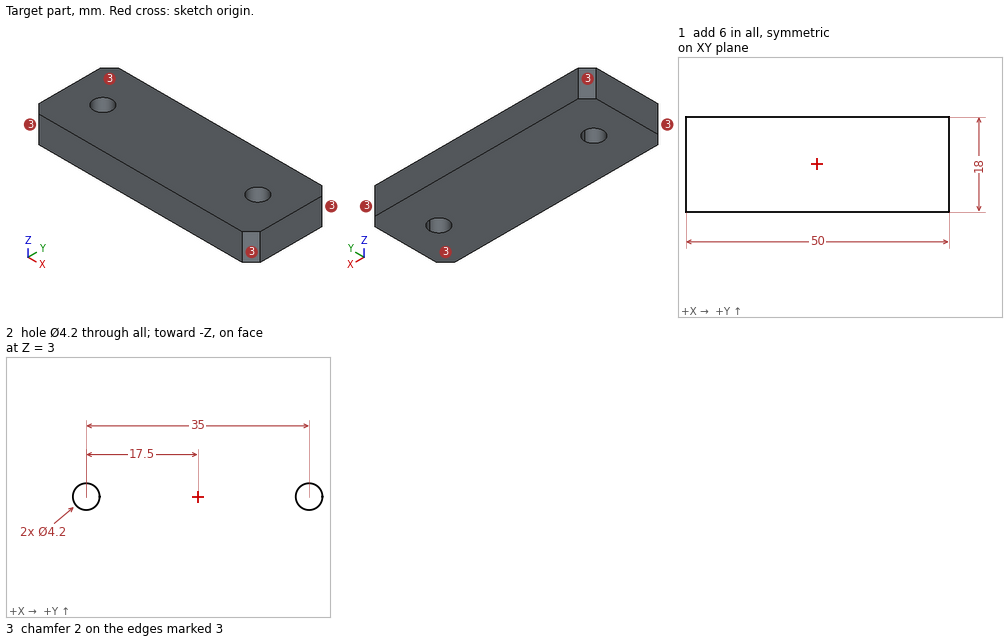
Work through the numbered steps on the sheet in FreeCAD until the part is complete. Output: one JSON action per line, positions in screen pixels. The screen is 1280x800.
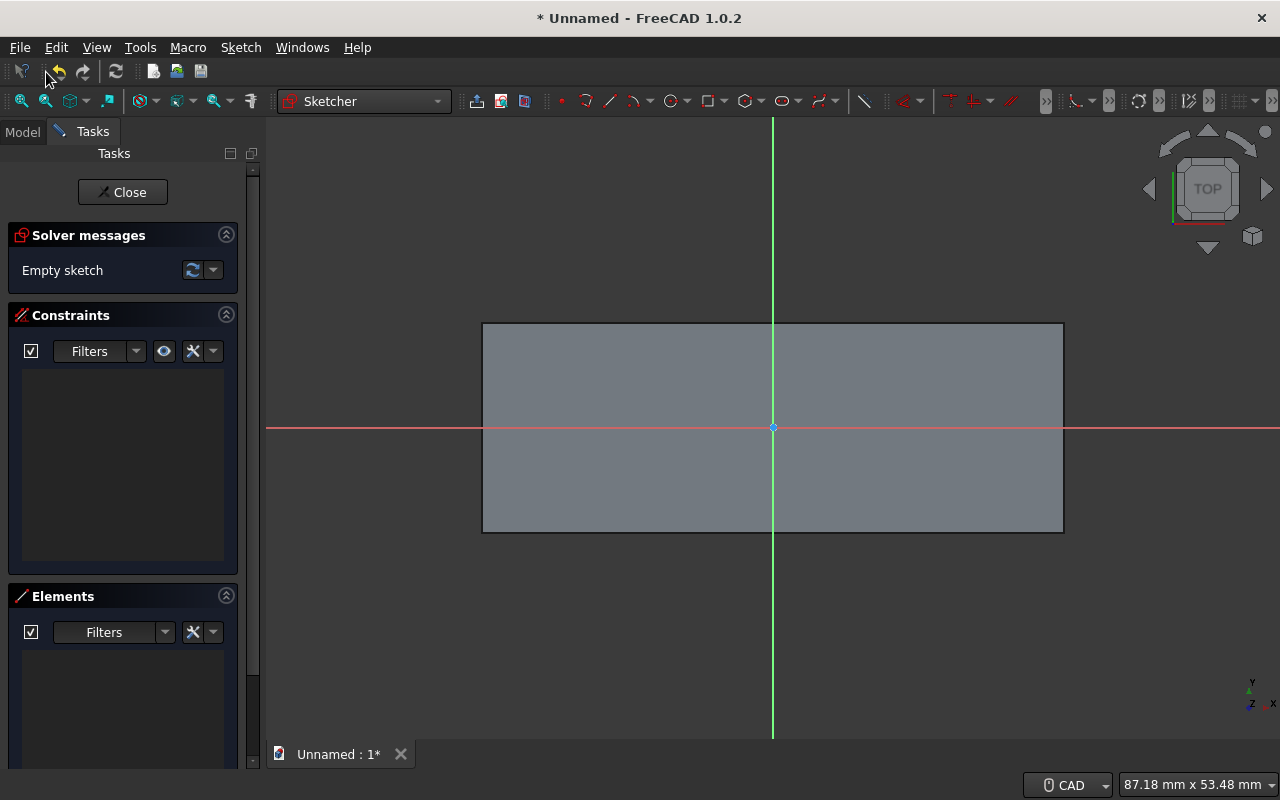
{"action": "key", "text": "g c"}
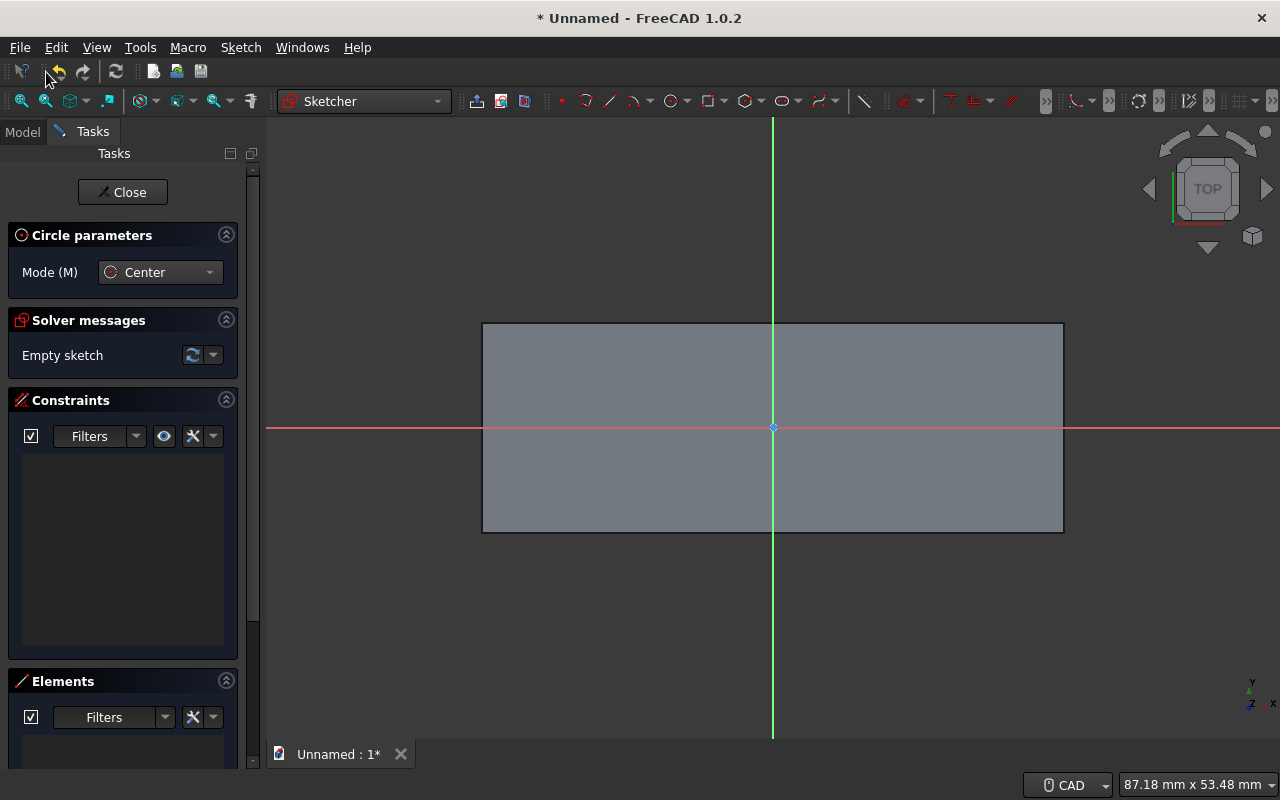
{"action": "left_click", "coordinate": [569, 428]}
{"action": "left_click", "coordinate": [587, 411]}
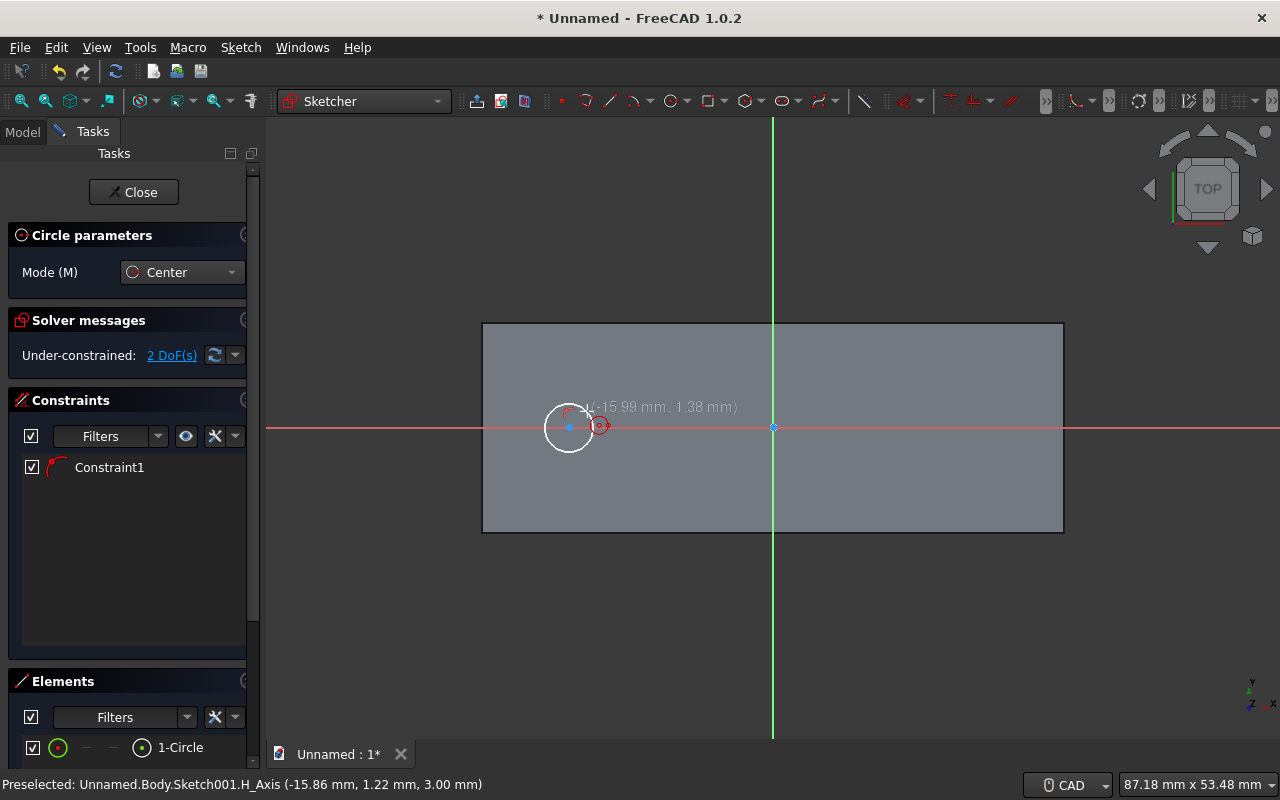
{"action": "left_click", "coordinate": [977, 428]}
{"action": "left_click", "coordinate": [994, 411]}
{"action": "key", "text": "Escape"}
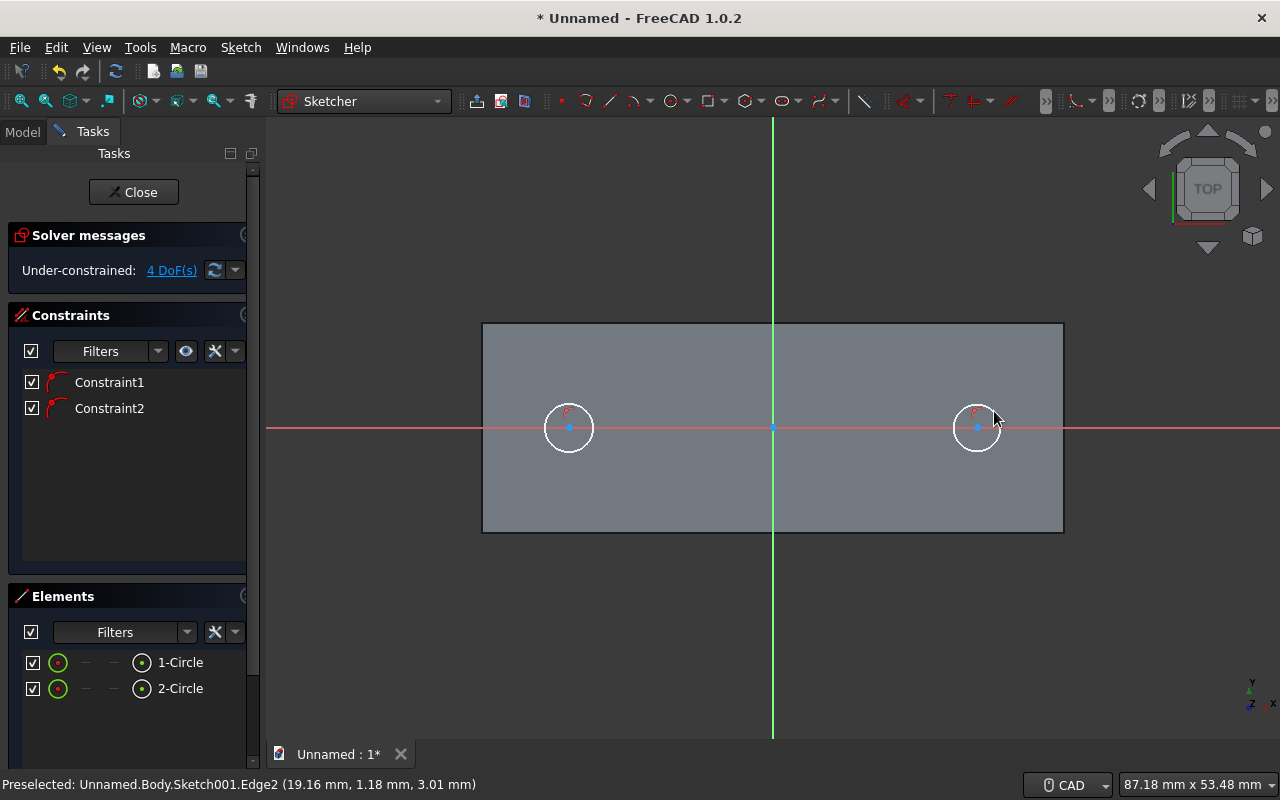
{"action": "left_click", "coordinate": [586, 411]}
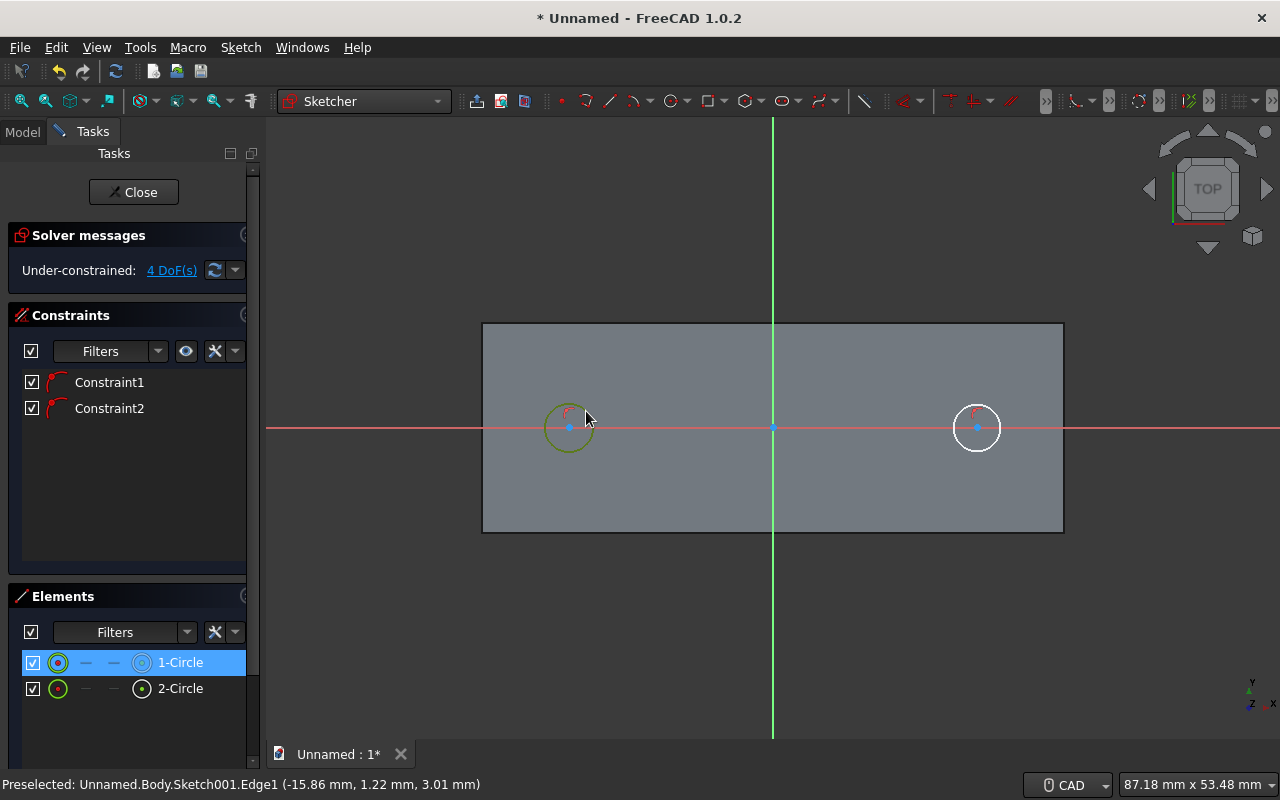
{"action": "left_click", "coordinate": [993, 411]}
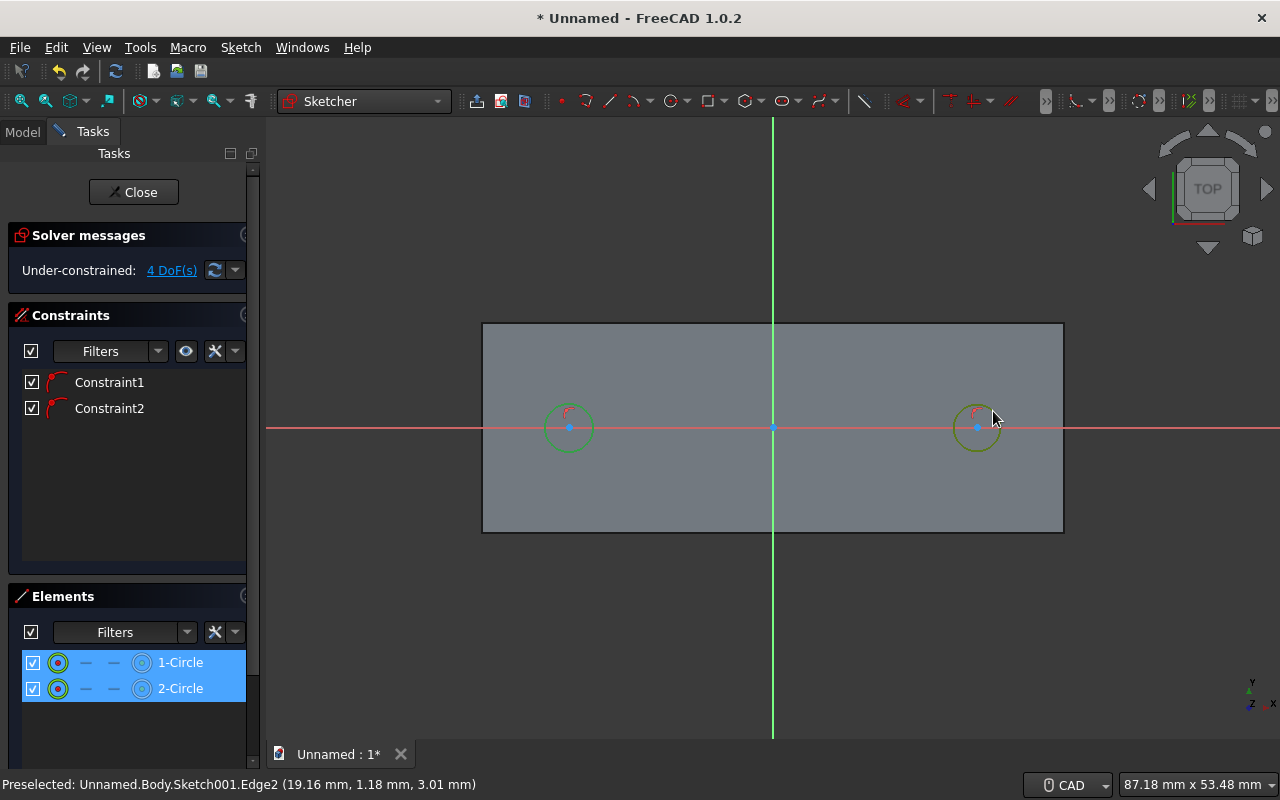
{"action": "key", "text": "e"}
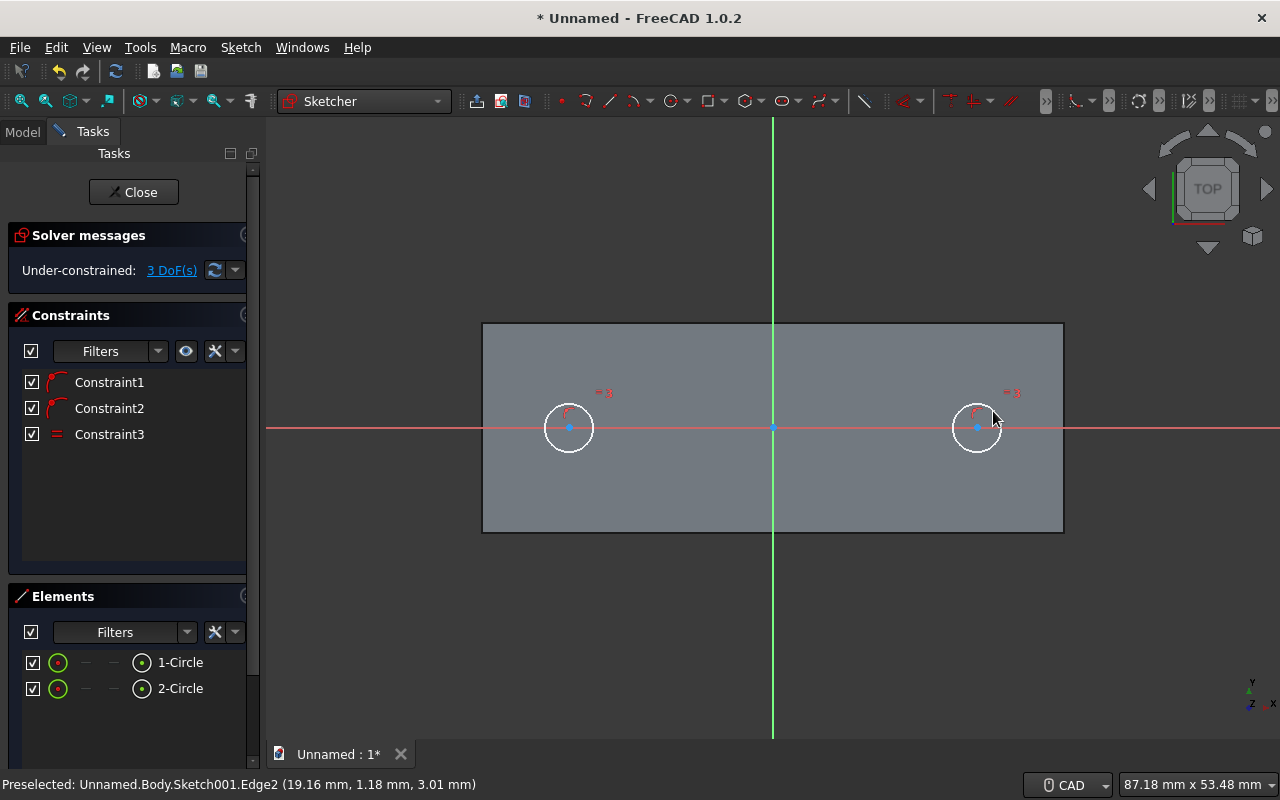
{"action": "key", "text": "d"}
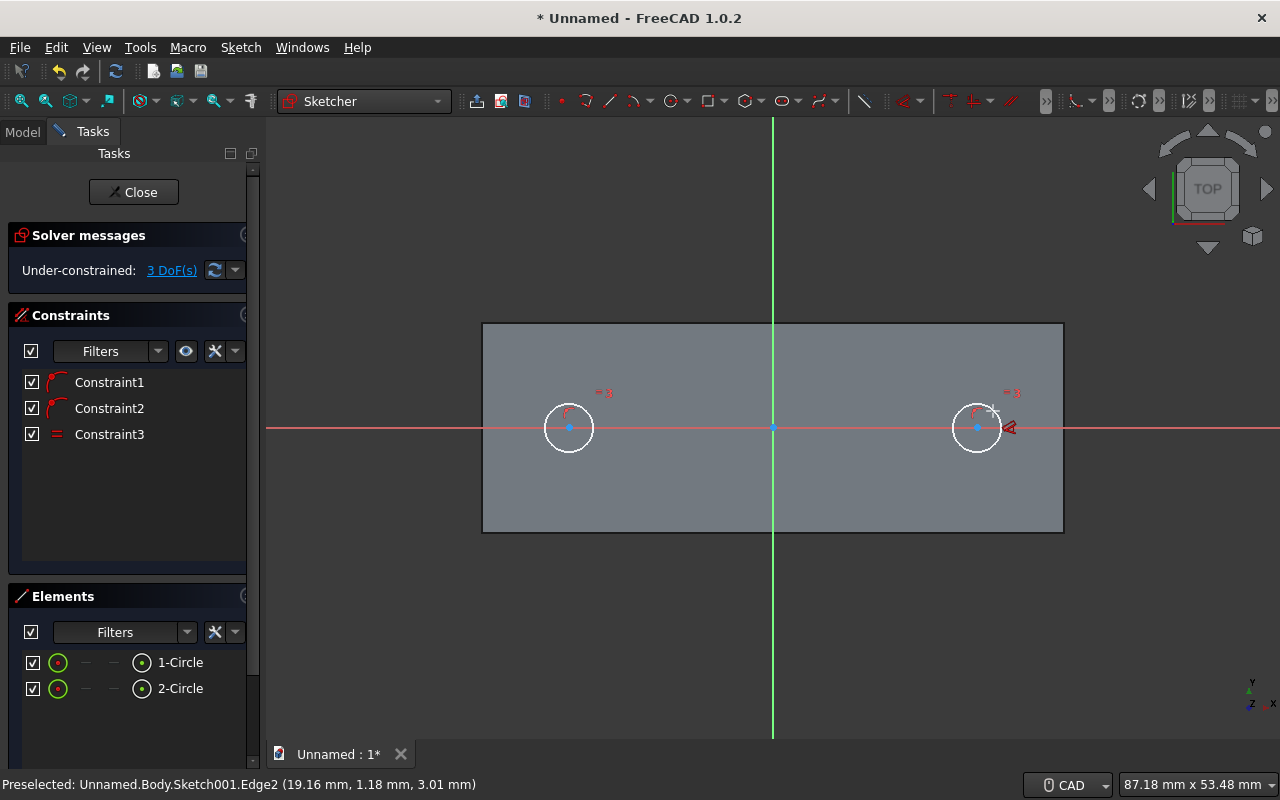
{"action": "left_click", "coordinate": [586, 411]}
{"action": "left_click", "coordinate": [609, 388]}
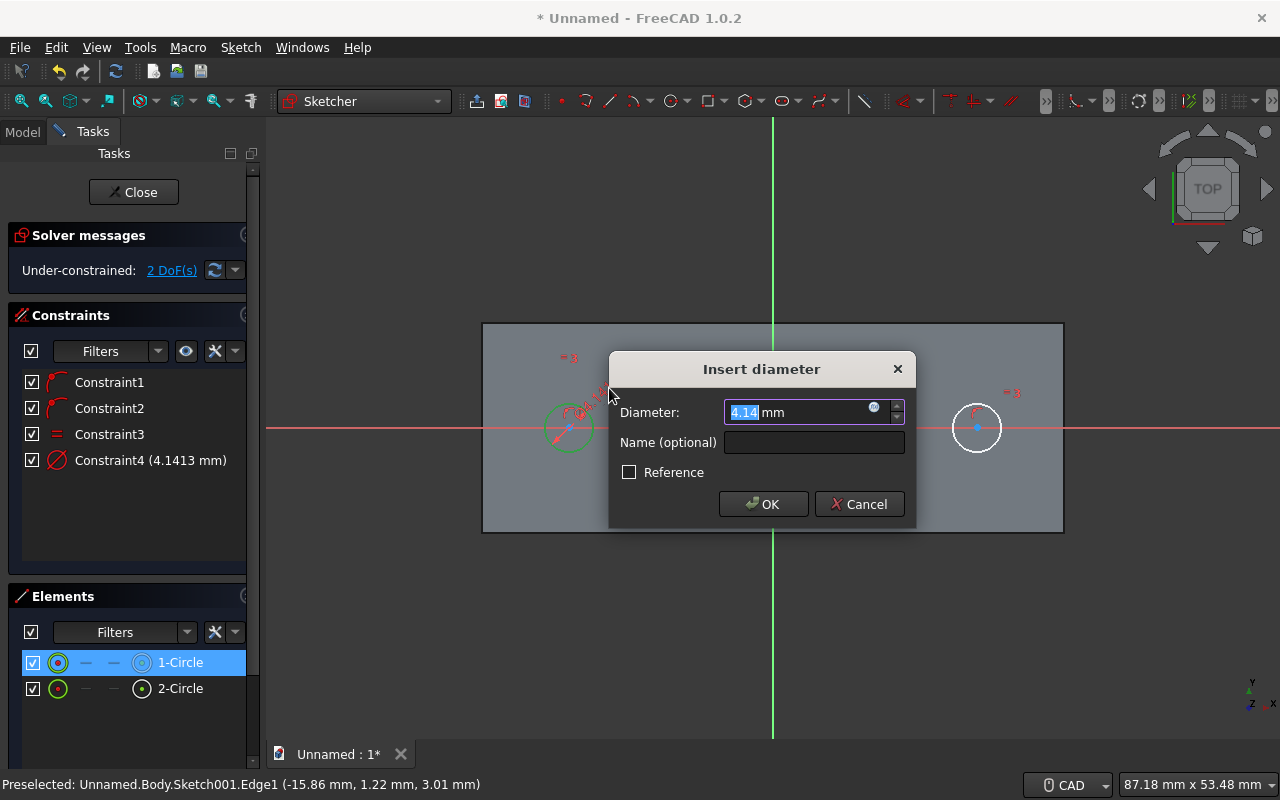
{"action": "type", "text": "4.2"}
{"action": "key", "text": "Return"}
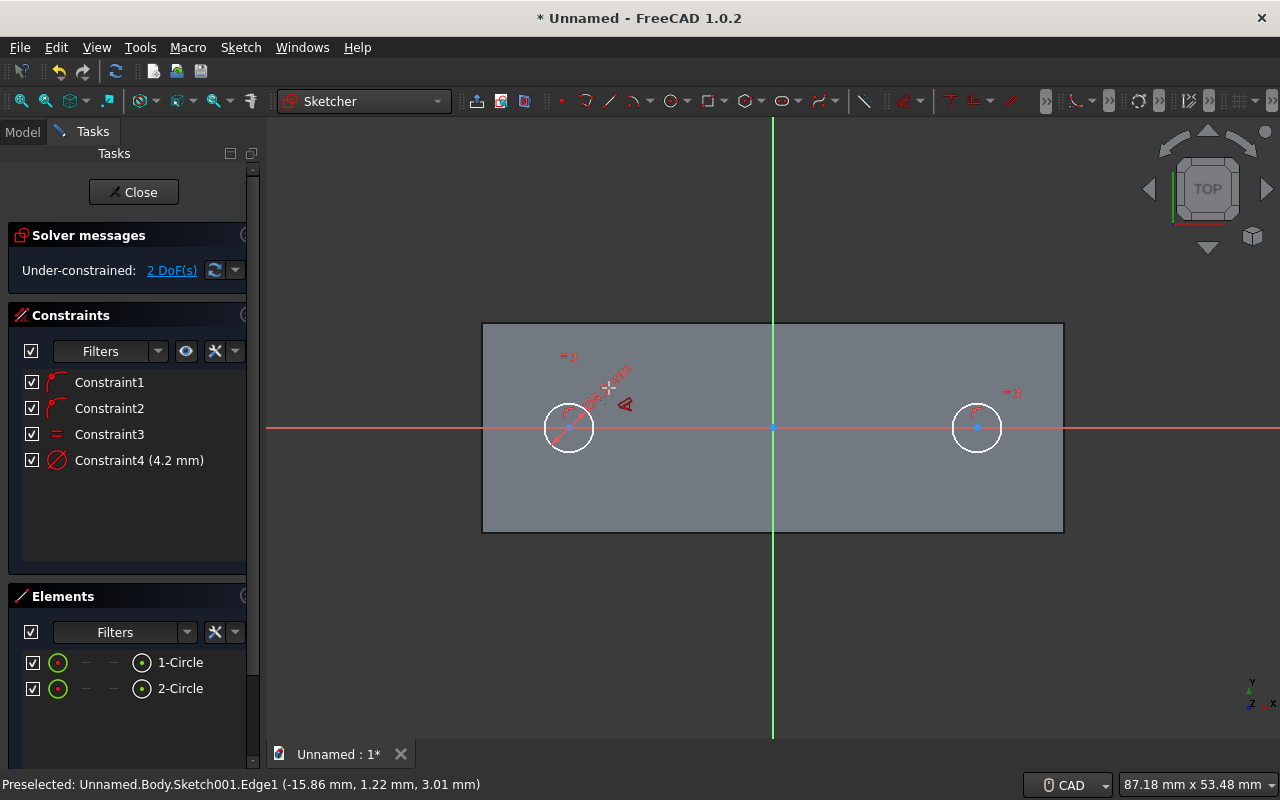
{"action": "left_click", "coordinate": [569, 428]}